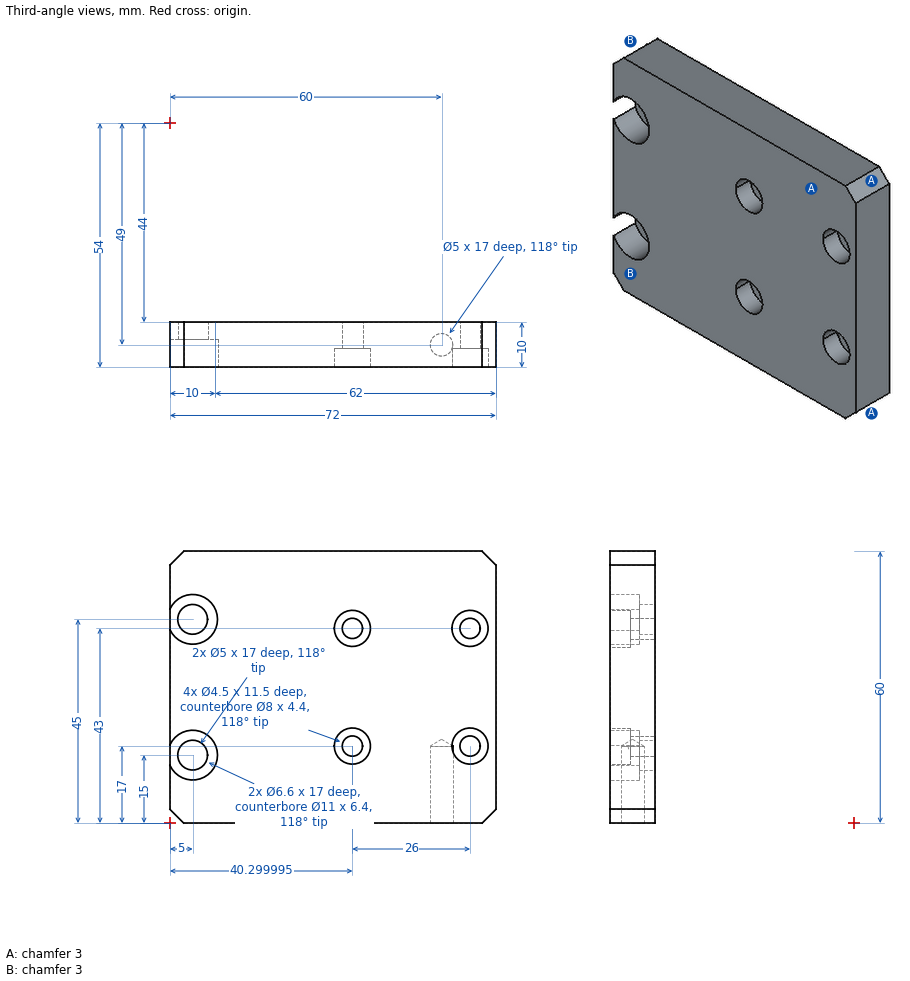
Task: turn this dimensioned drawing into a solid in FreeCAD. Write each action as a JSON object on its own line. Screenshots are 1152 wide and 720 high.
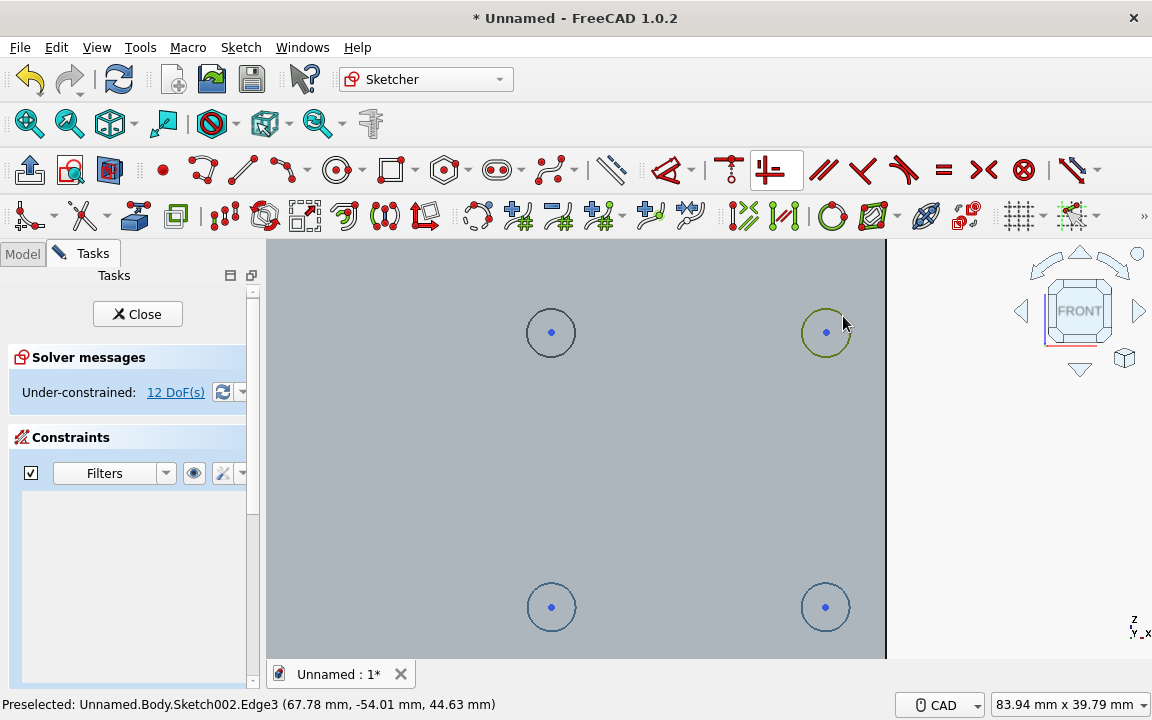
{"action": "left_click", "coordinate": [568, 316]}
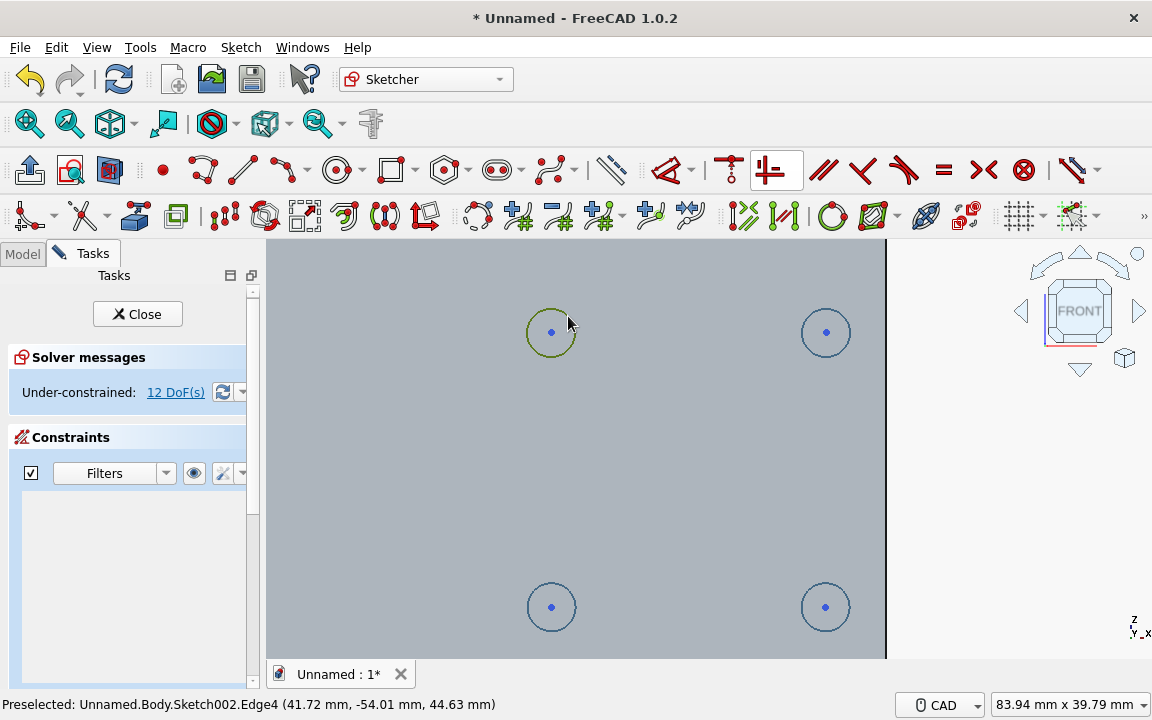
{"action": "left_click", "coordinate": [944, 170]}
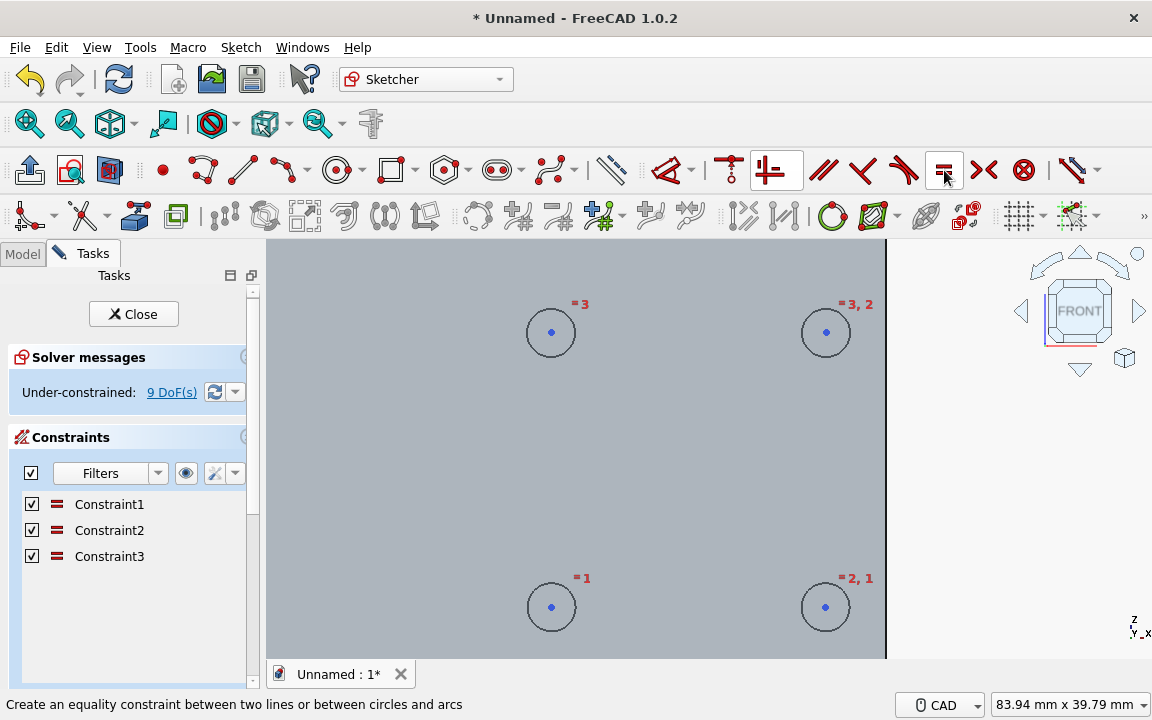
{"action": "left_click", "coordinate": [552, 607]}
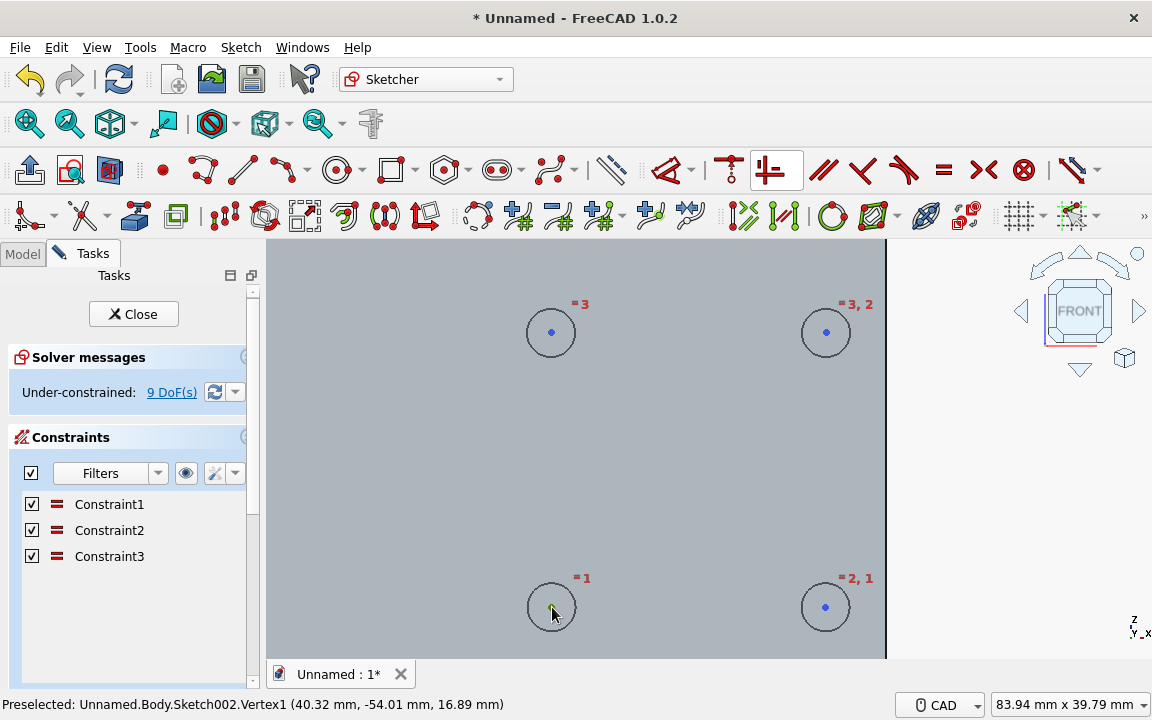
{"action": "left_click", "coordinate": [826, 607]}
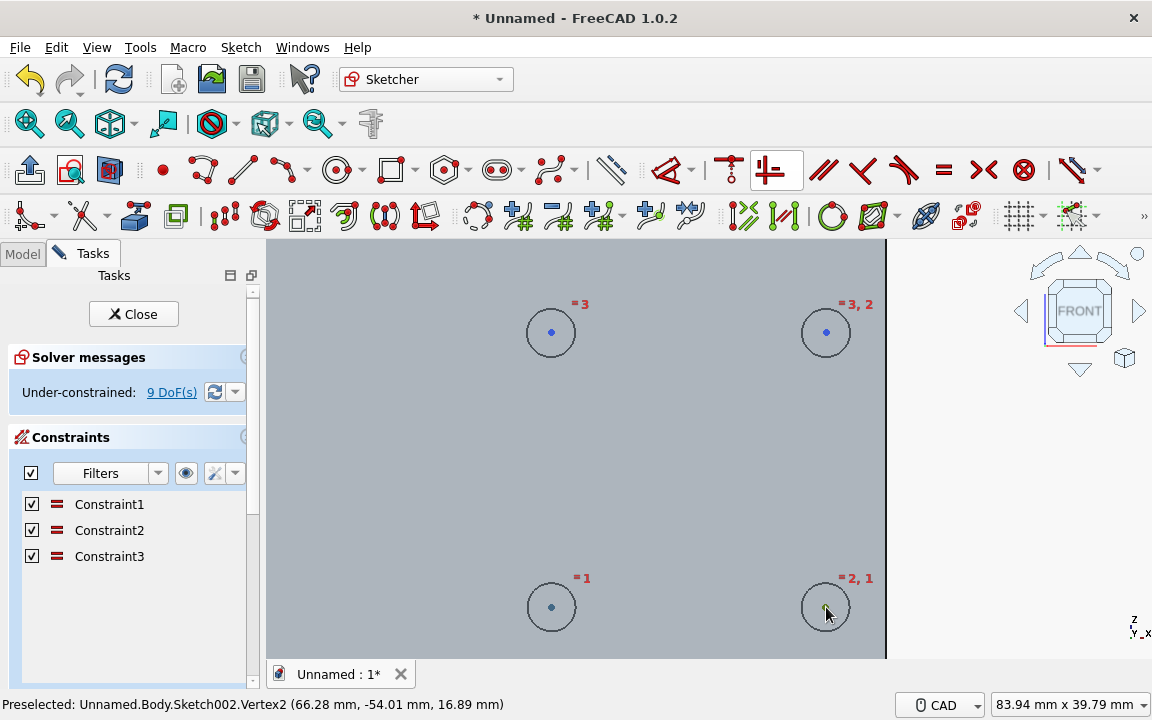
{"action": "key", "text": "h"}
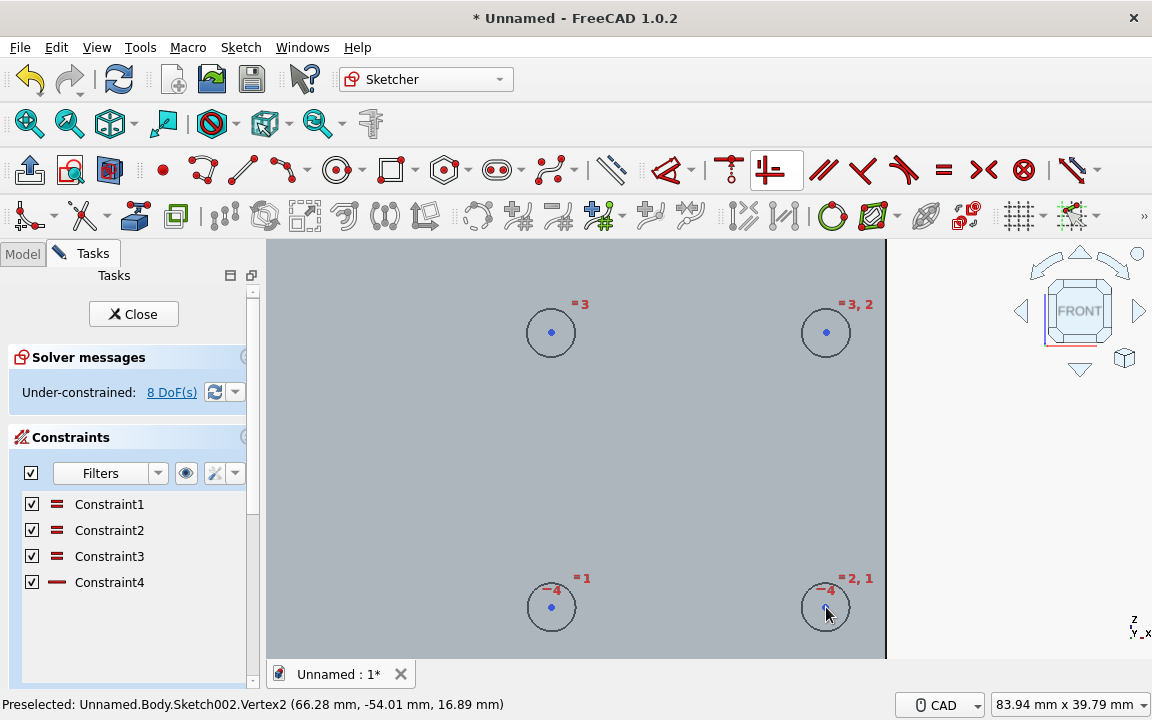
{"action": "left_click", "coordinate": [826, 607]}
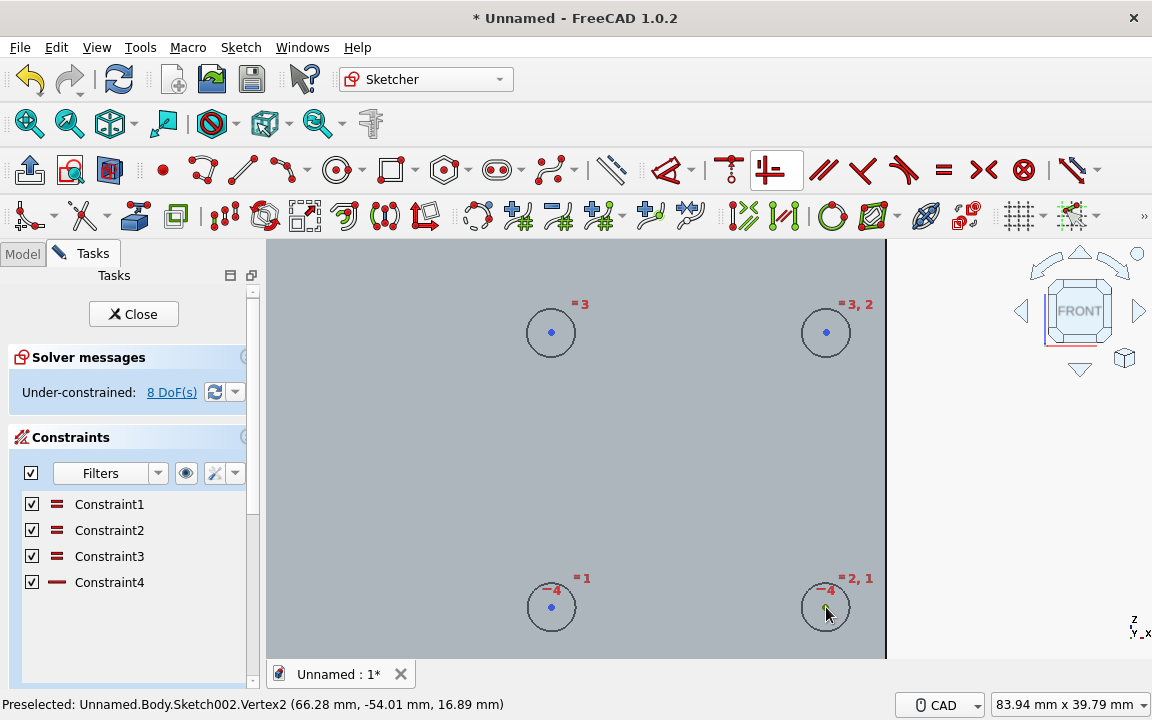
{"action": "left_click", "coordinate": [826, 333]}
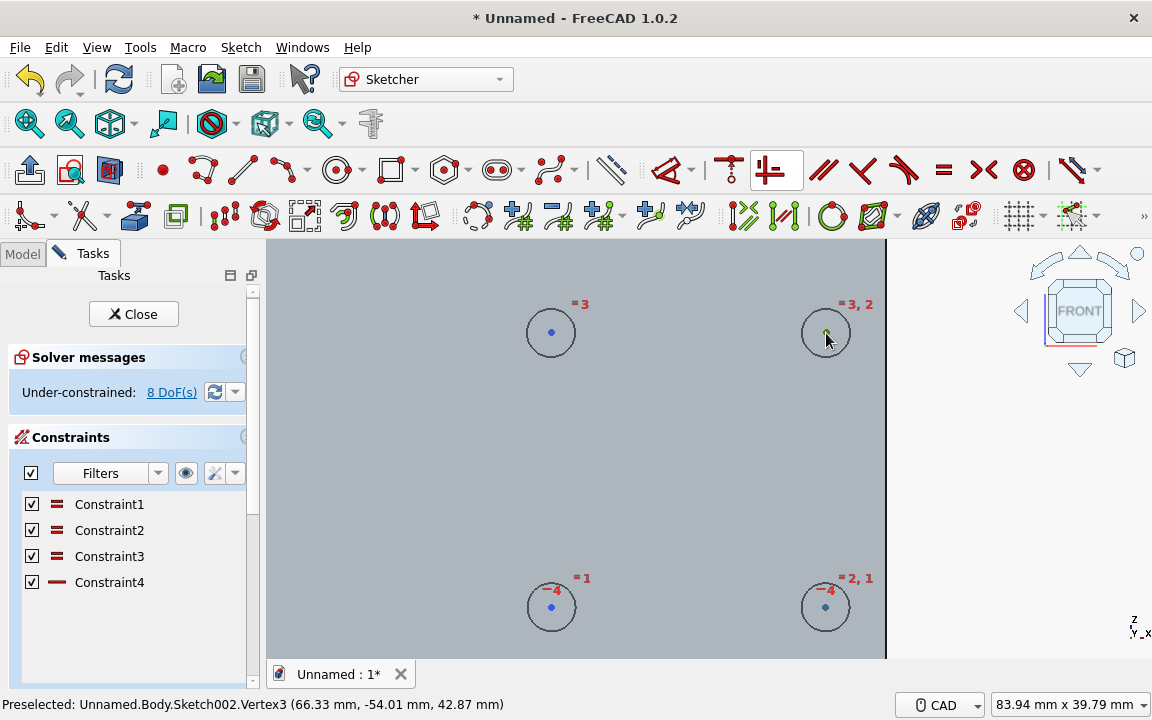
{"action": "left_click", "coordinate": [798, 170]}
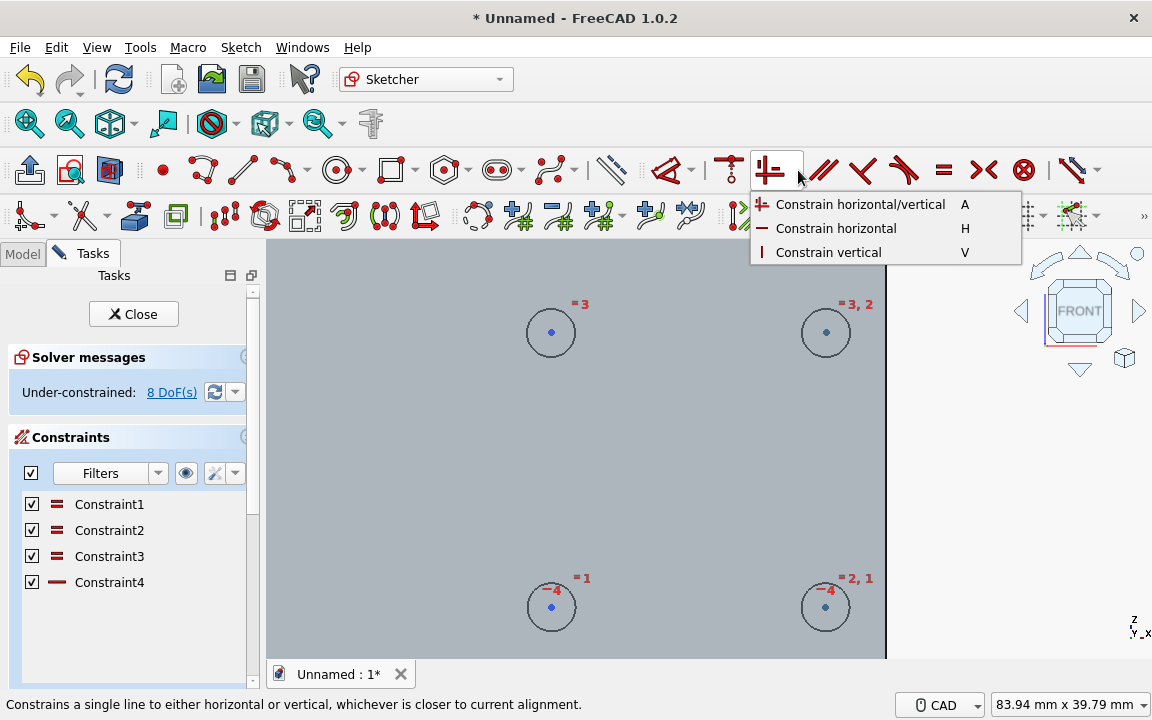
{"action": "left_click", "coordinate": [886, 252]}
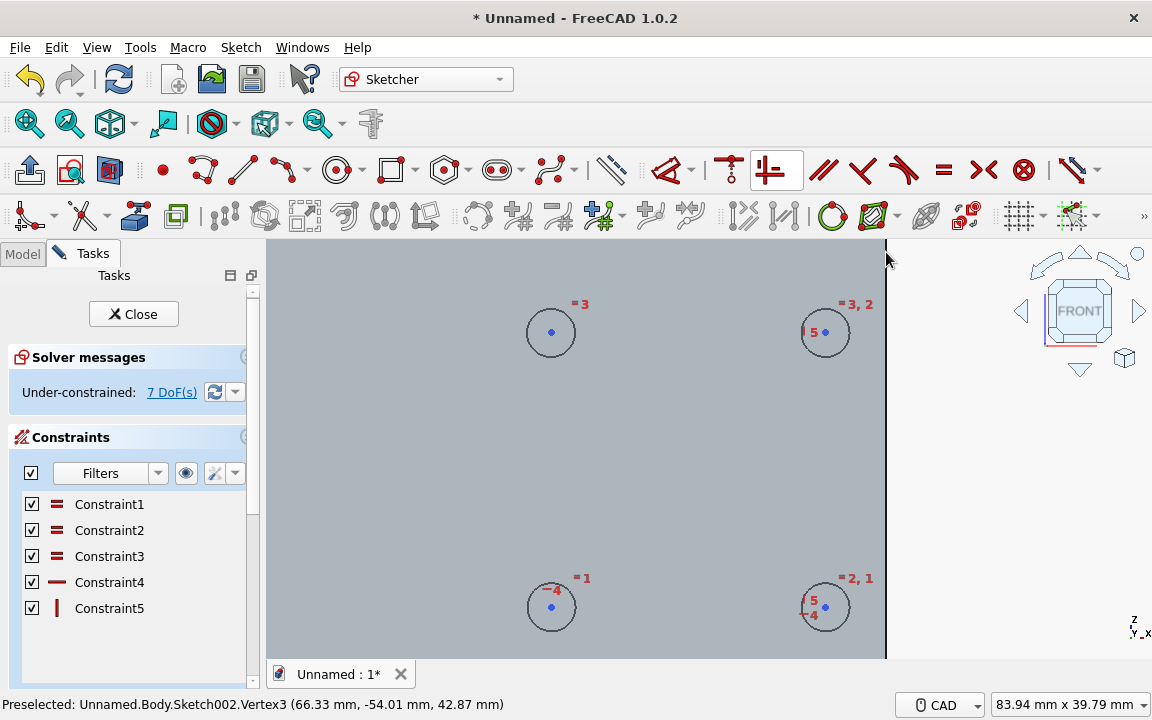
{"action": "left_click", "coordinate": [552, 607]}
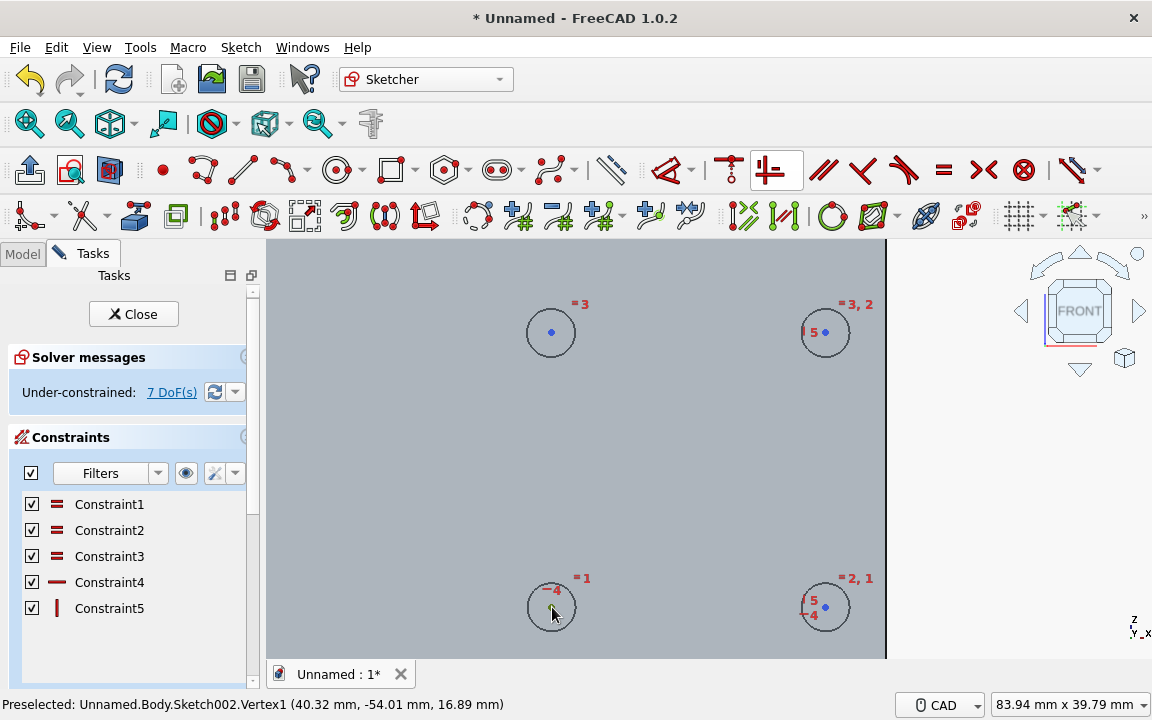
{"action": "left_click", "coordinate": [551, 333]}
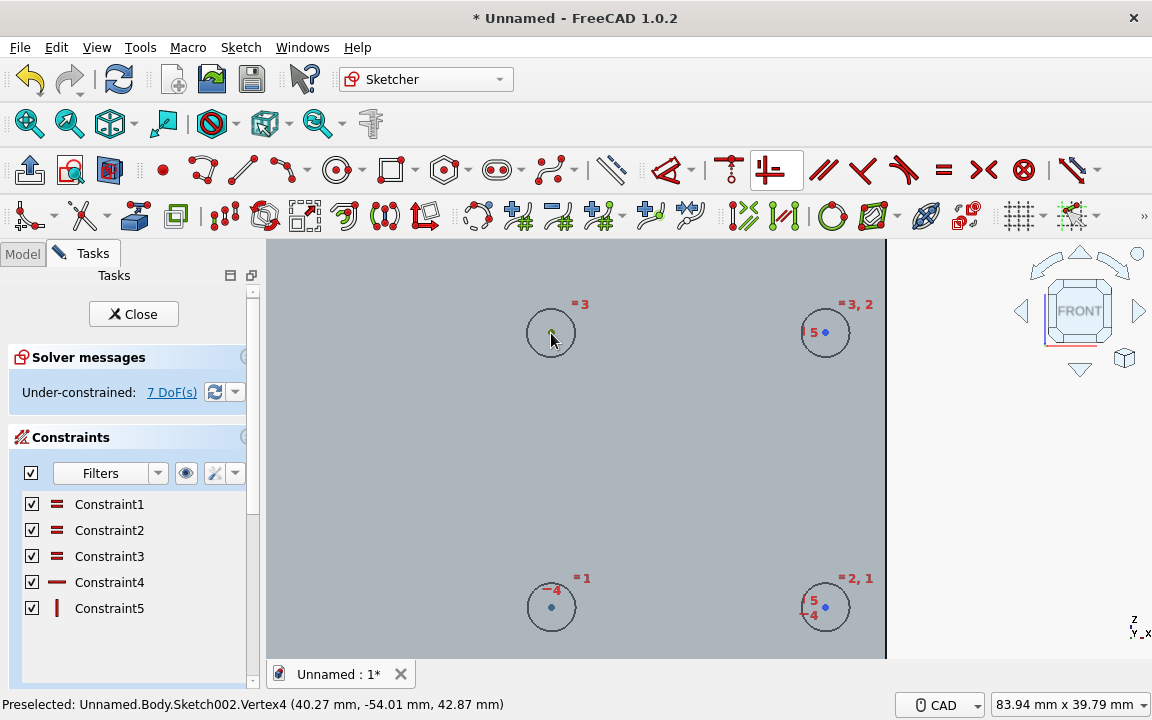
{"action": "left_click", "coordinate": [798, 170]}